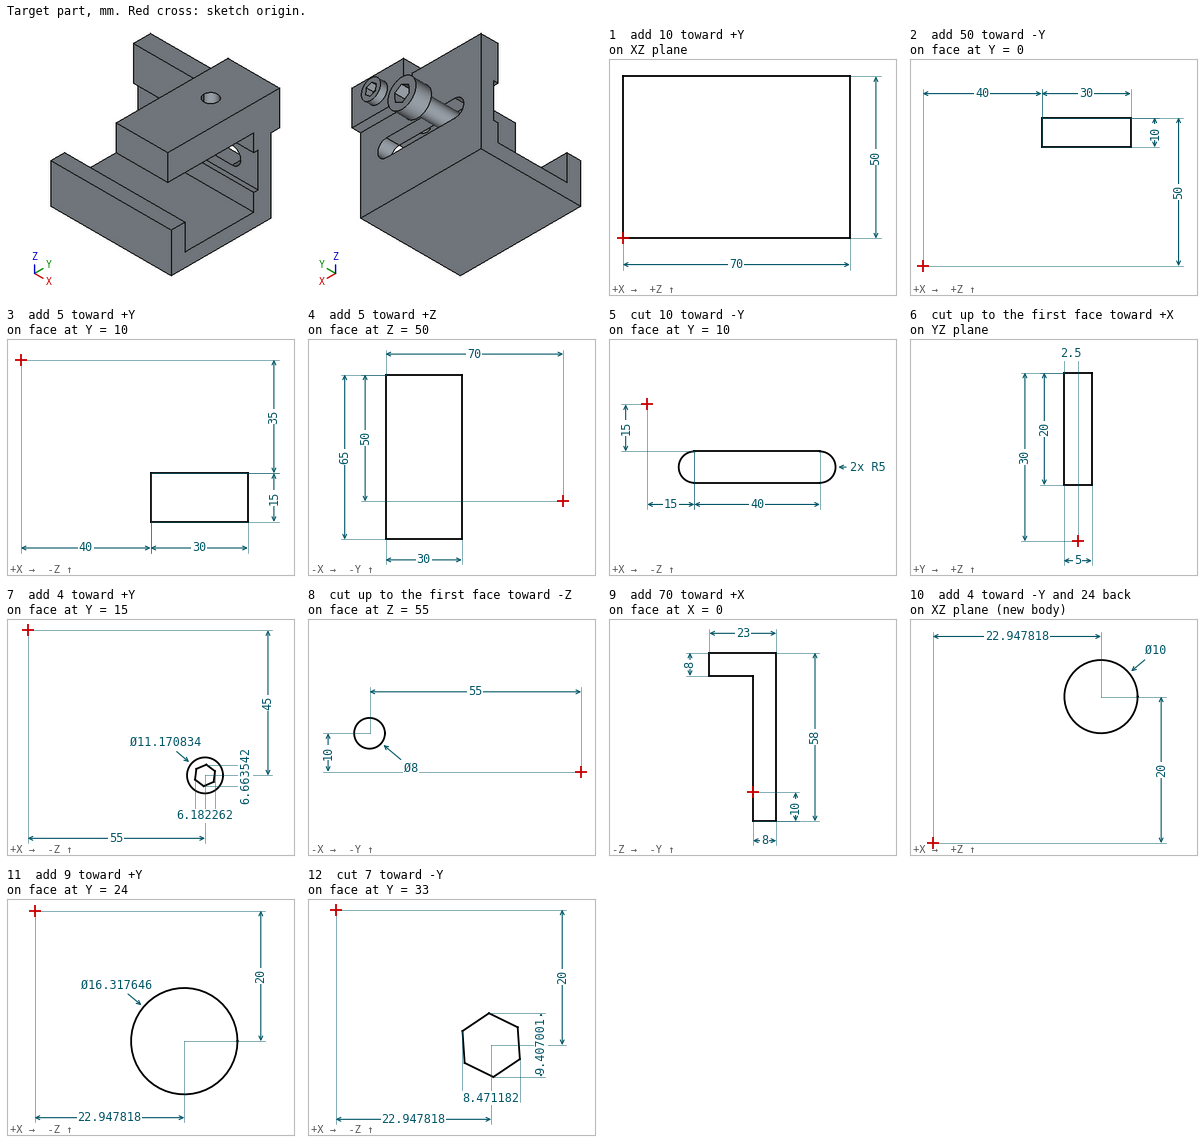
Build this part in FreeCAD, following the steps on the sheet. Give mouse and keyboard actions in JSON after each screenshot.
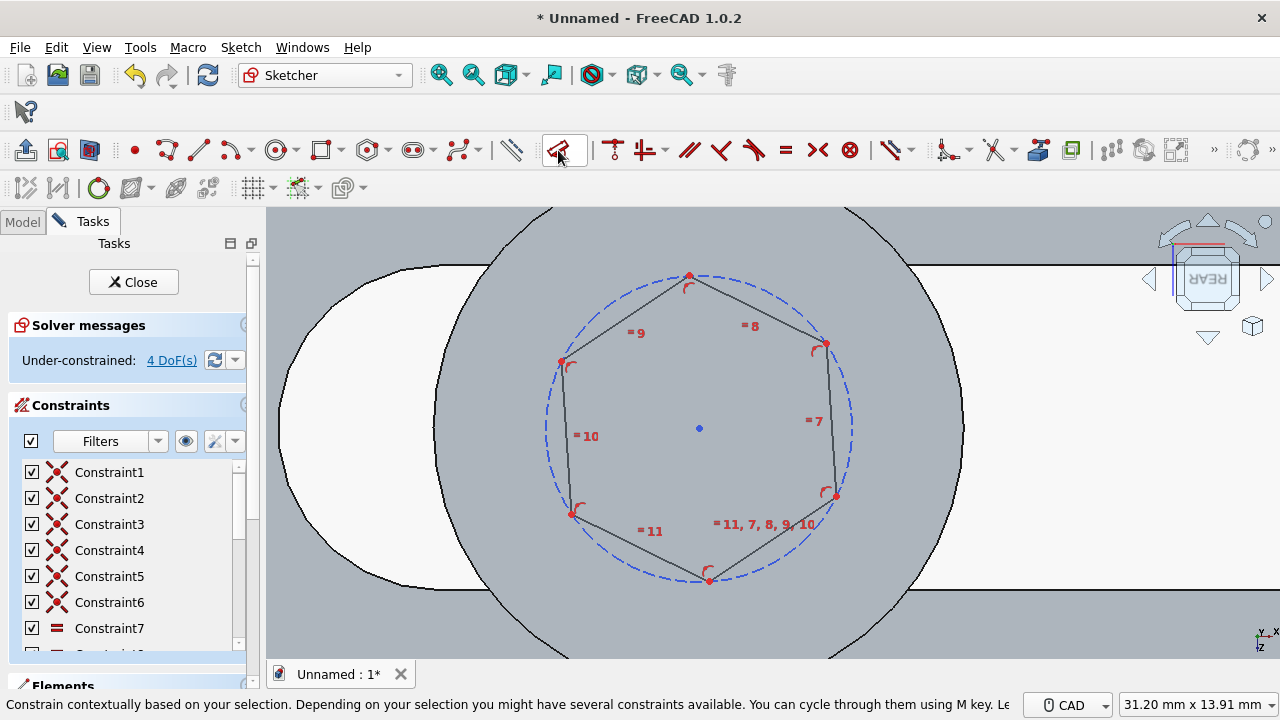
{"action": "left_click", "coordinate": [699, 429]}
{"action": "left_click", "coordinate": [733, 332]}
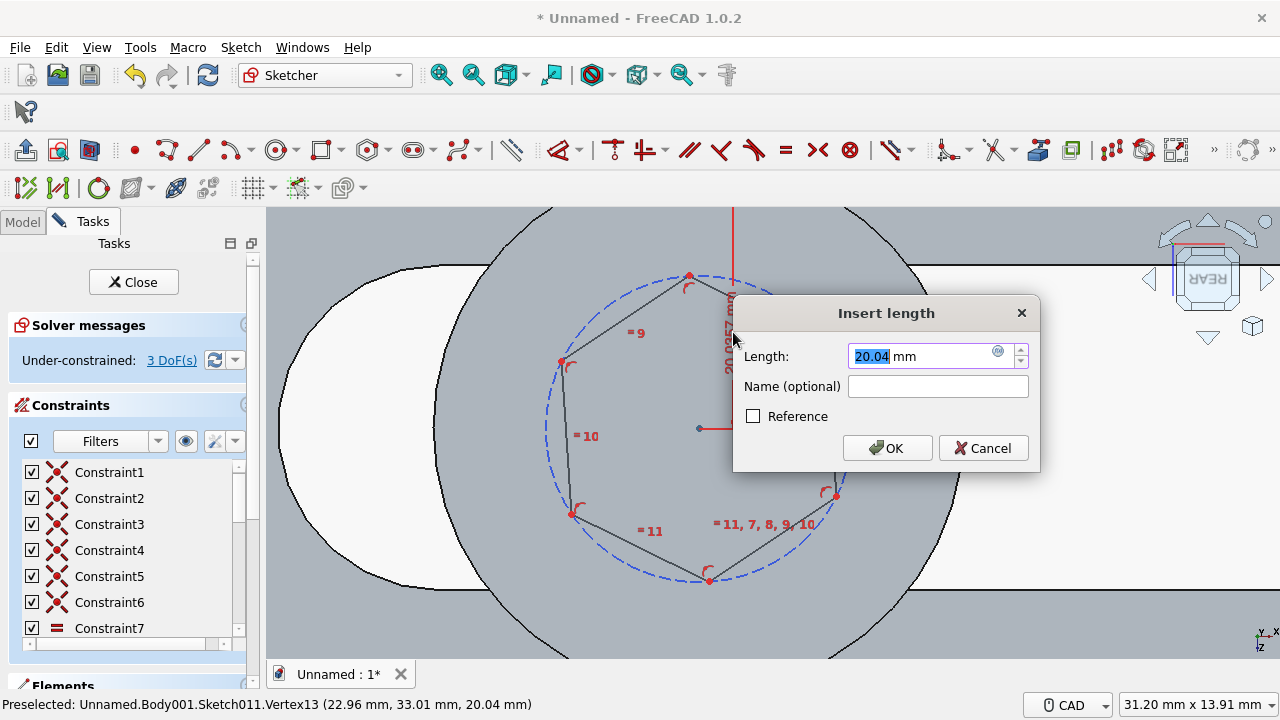
{"action": "type", "text": "20"}
{"action": "key", "text": "Return"}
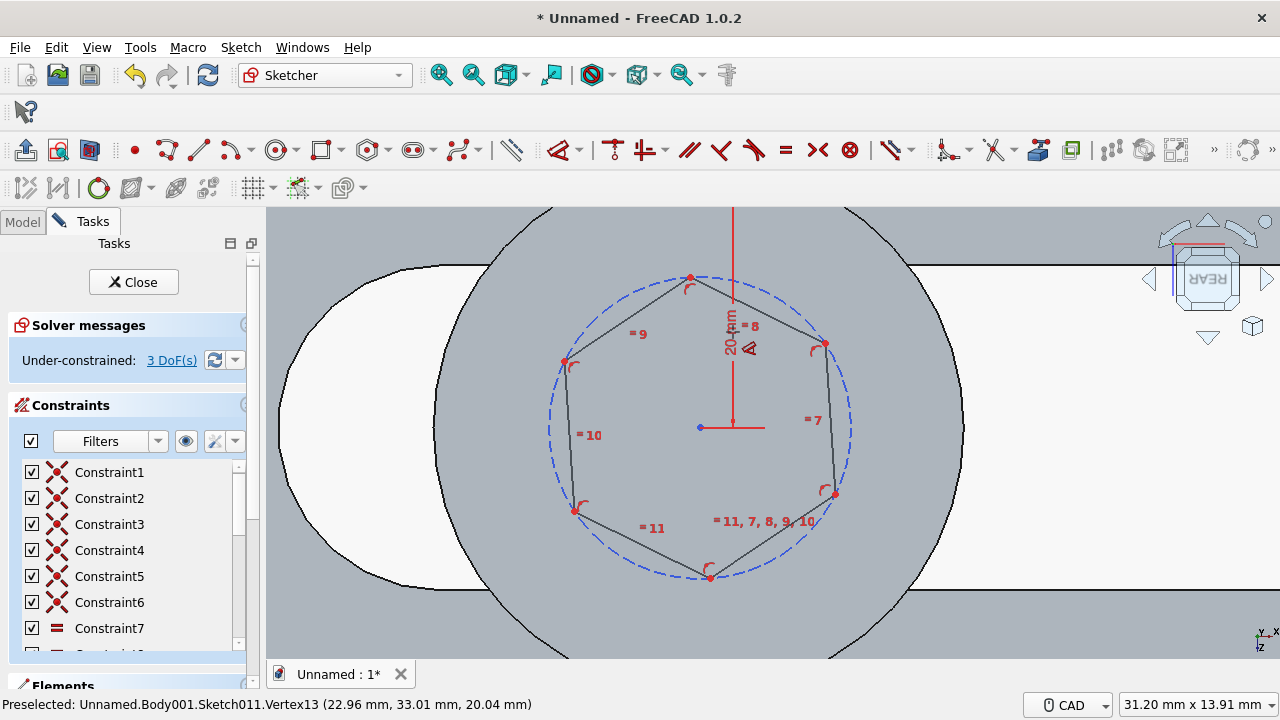
{"action": "left_click", "coordinate": [710, 579]}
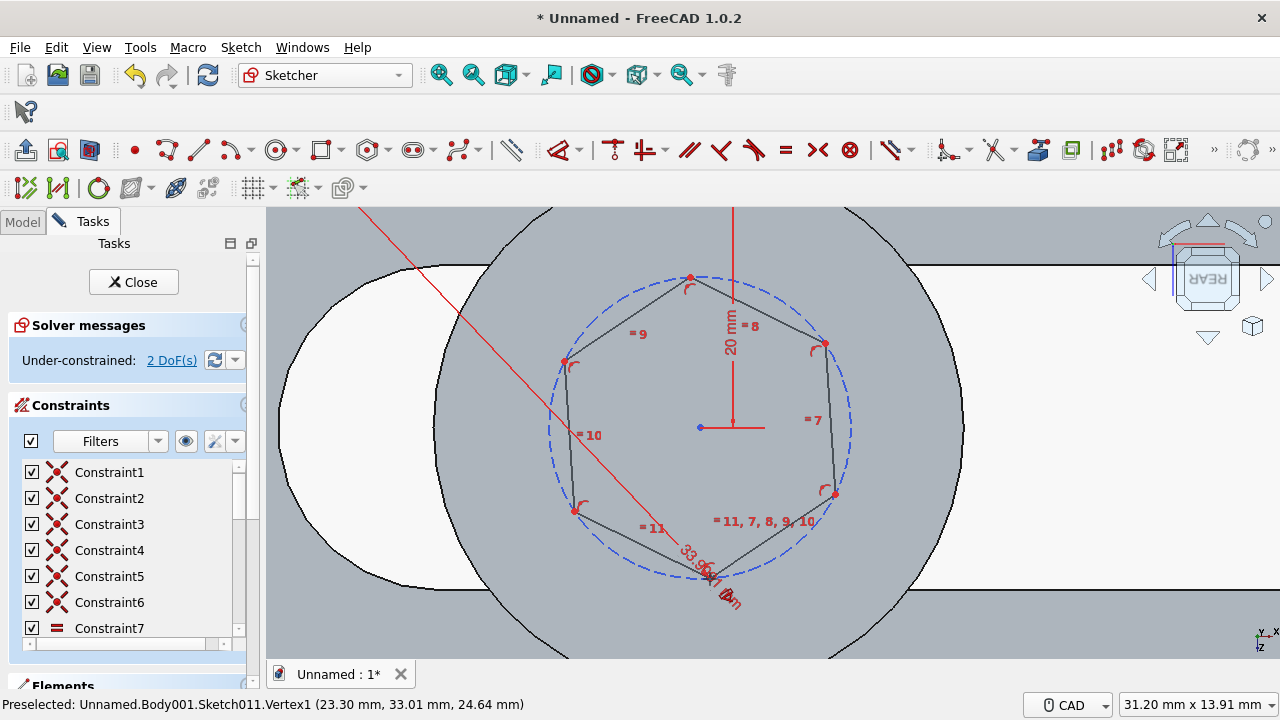
{"action": "left_click", "coordinate": [690, 277]}
{"action": "left_click", "coordinate": [744, 428]}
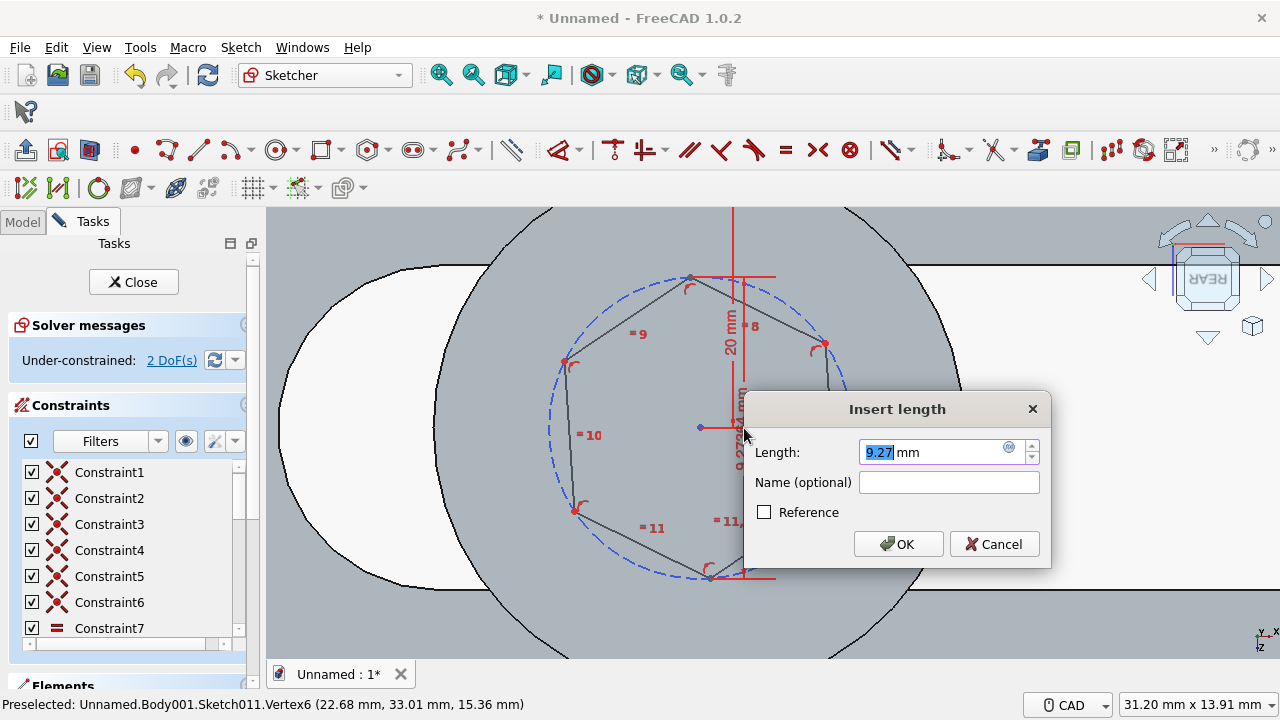
{"action": "type", "text": "9.407001"}
{"action": "key", "text": "Return"}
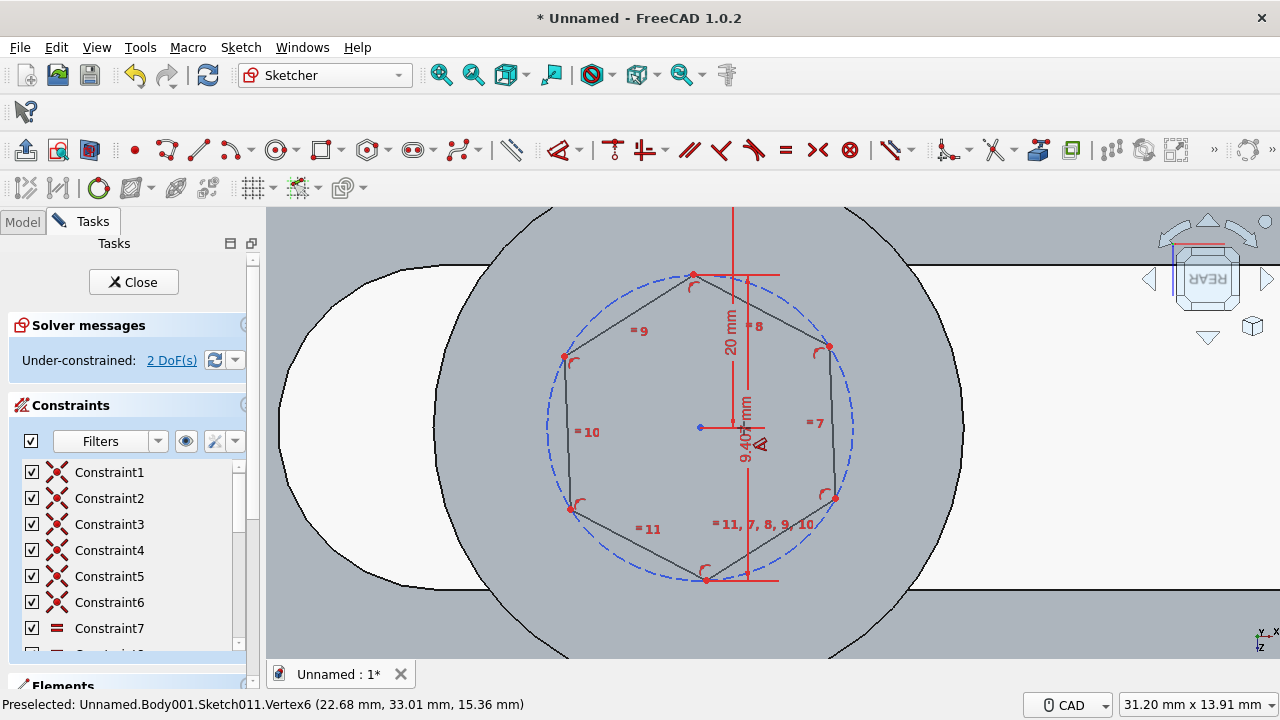
{"action": "left_click", "coordinate": [565, 357]}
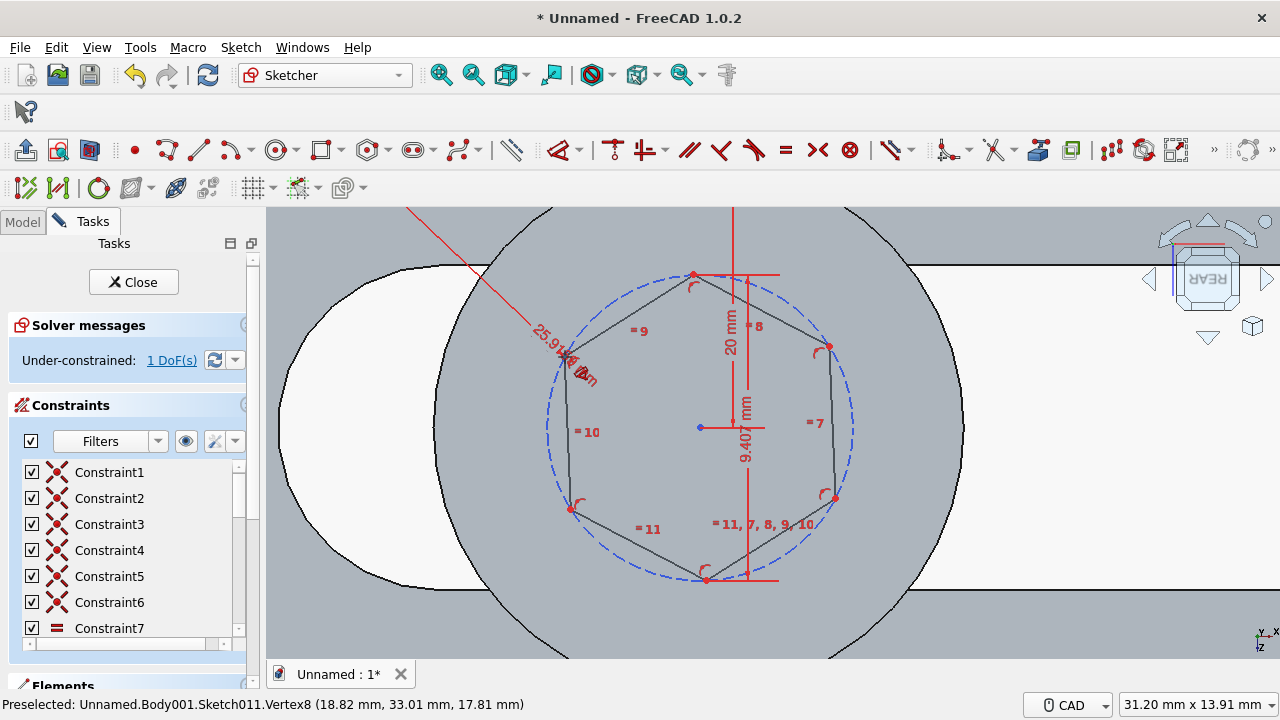
{"action": "left_click", "coordinate": [836, 499]}
{"action": "left_click", "coordinate": [700, 533]}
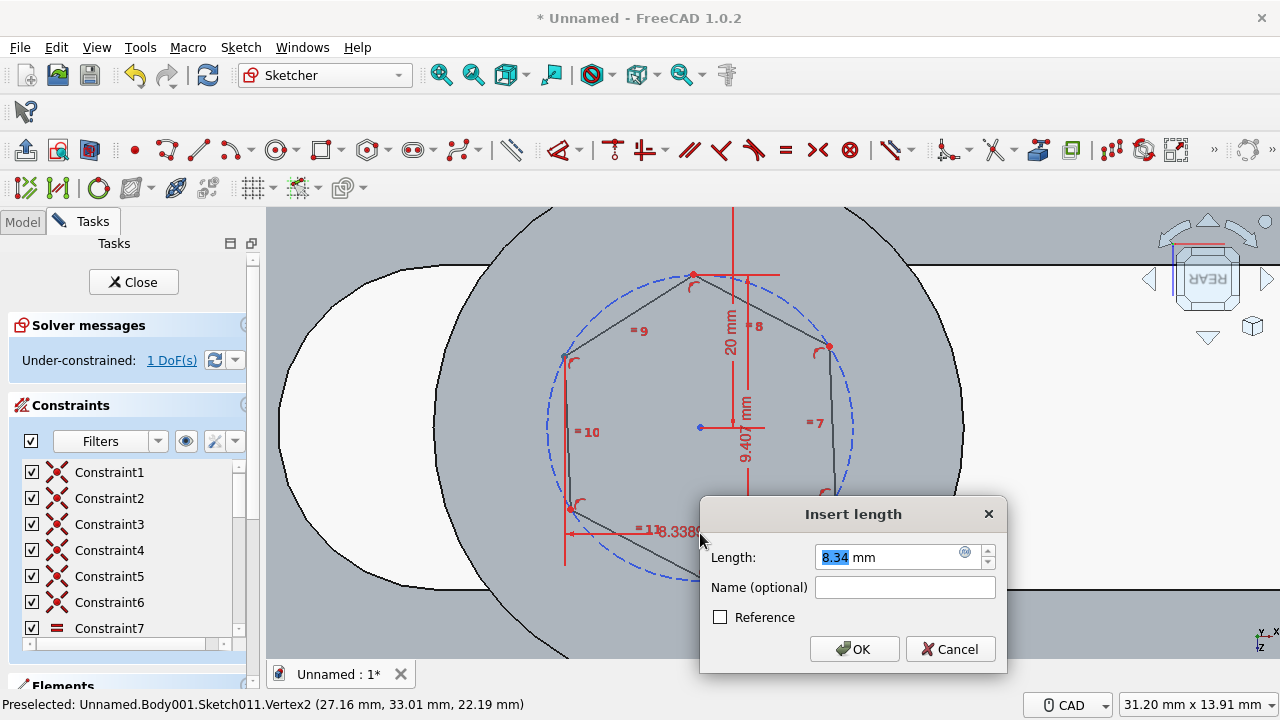
{"action": "type", "text": "8.471182"}
{"action": "key", "text": "Return"}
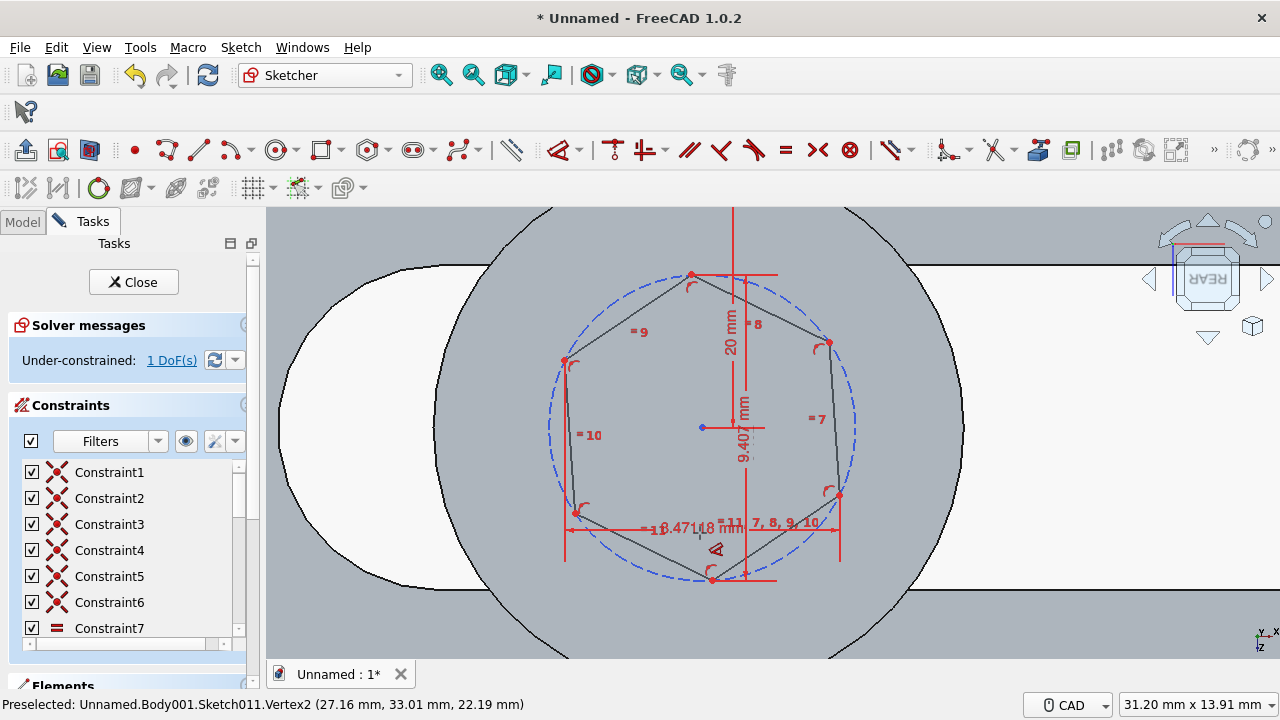
{"action": "left_click", "coordinate": [702, 428]}
{"action": "left_click", "coordinate": [498, 462]}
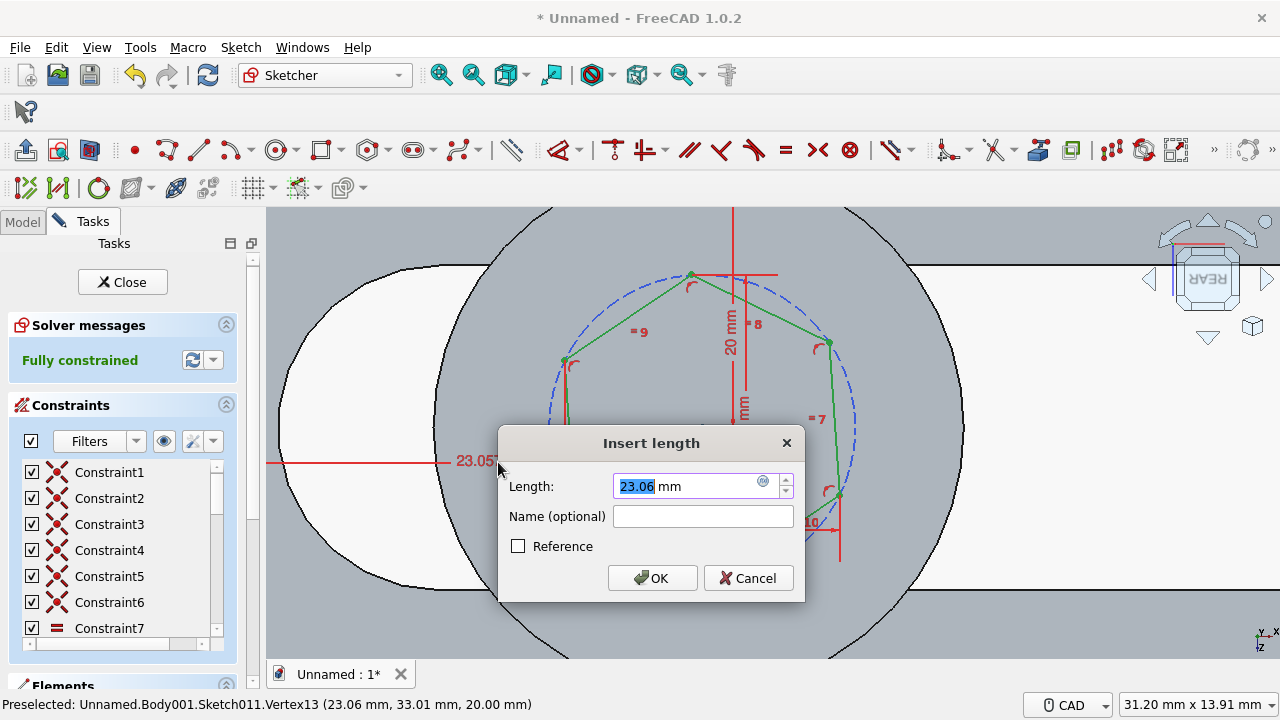
{"action": "type", "text": "22.947818"}
{"action": "key", "text": "Return"}
{"action": "key", "text": "Escape"}